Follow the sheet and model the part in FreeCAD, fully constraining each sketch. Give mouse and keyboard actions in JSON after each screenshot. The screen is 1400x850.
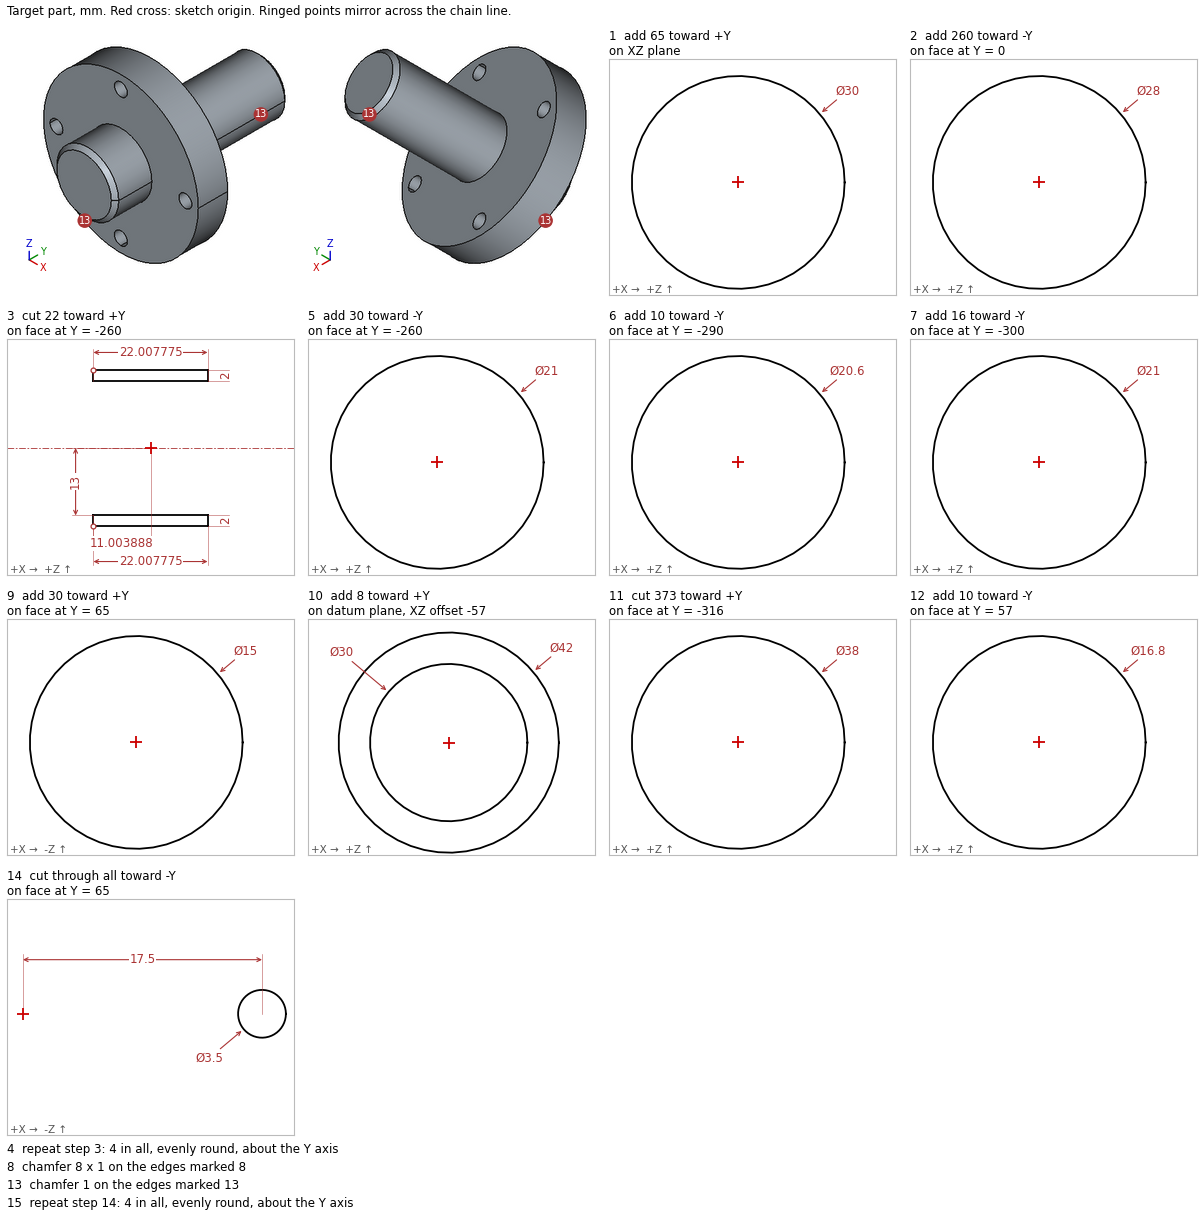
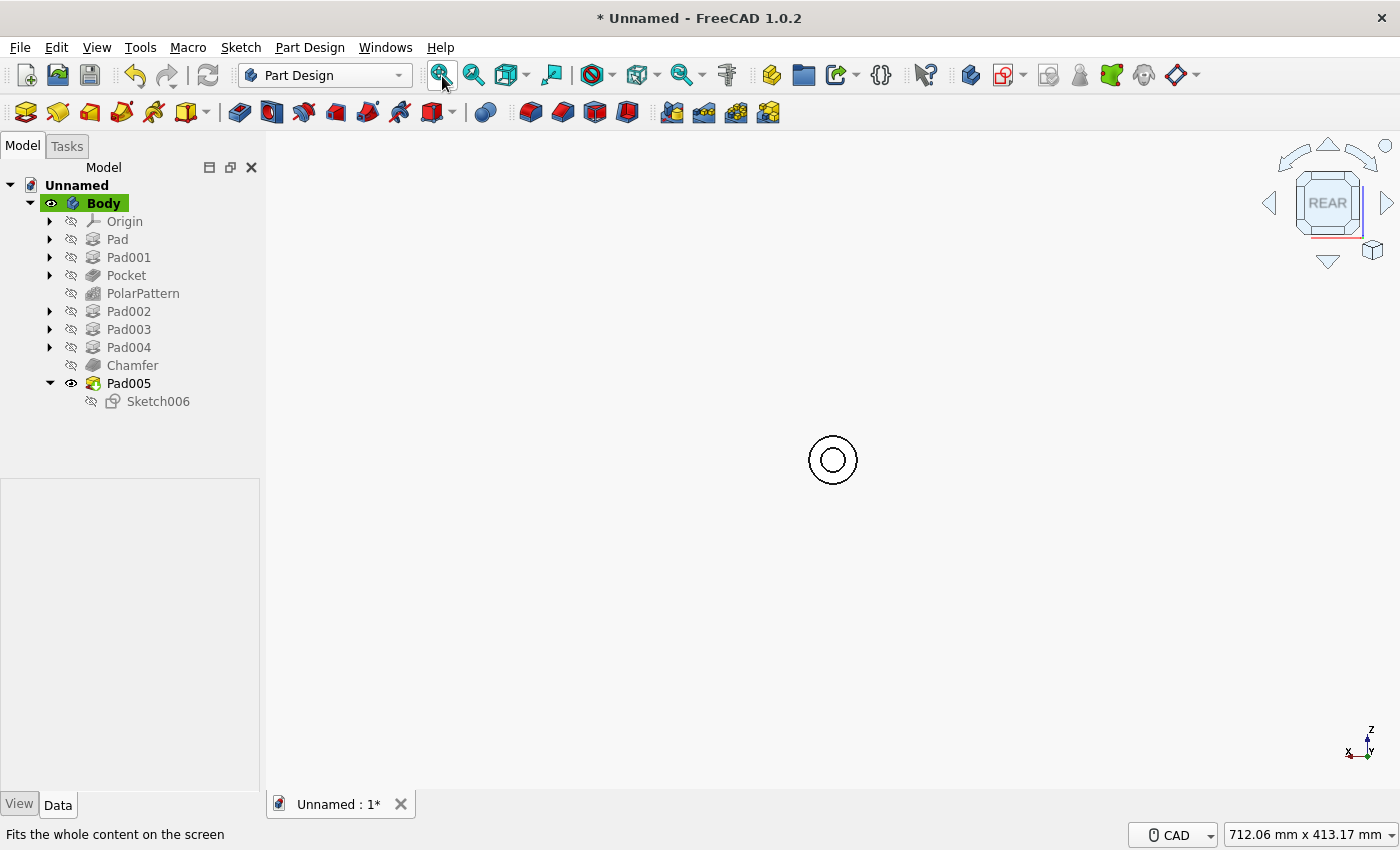
{"action": "left_click", "coordinate": [50, 221]}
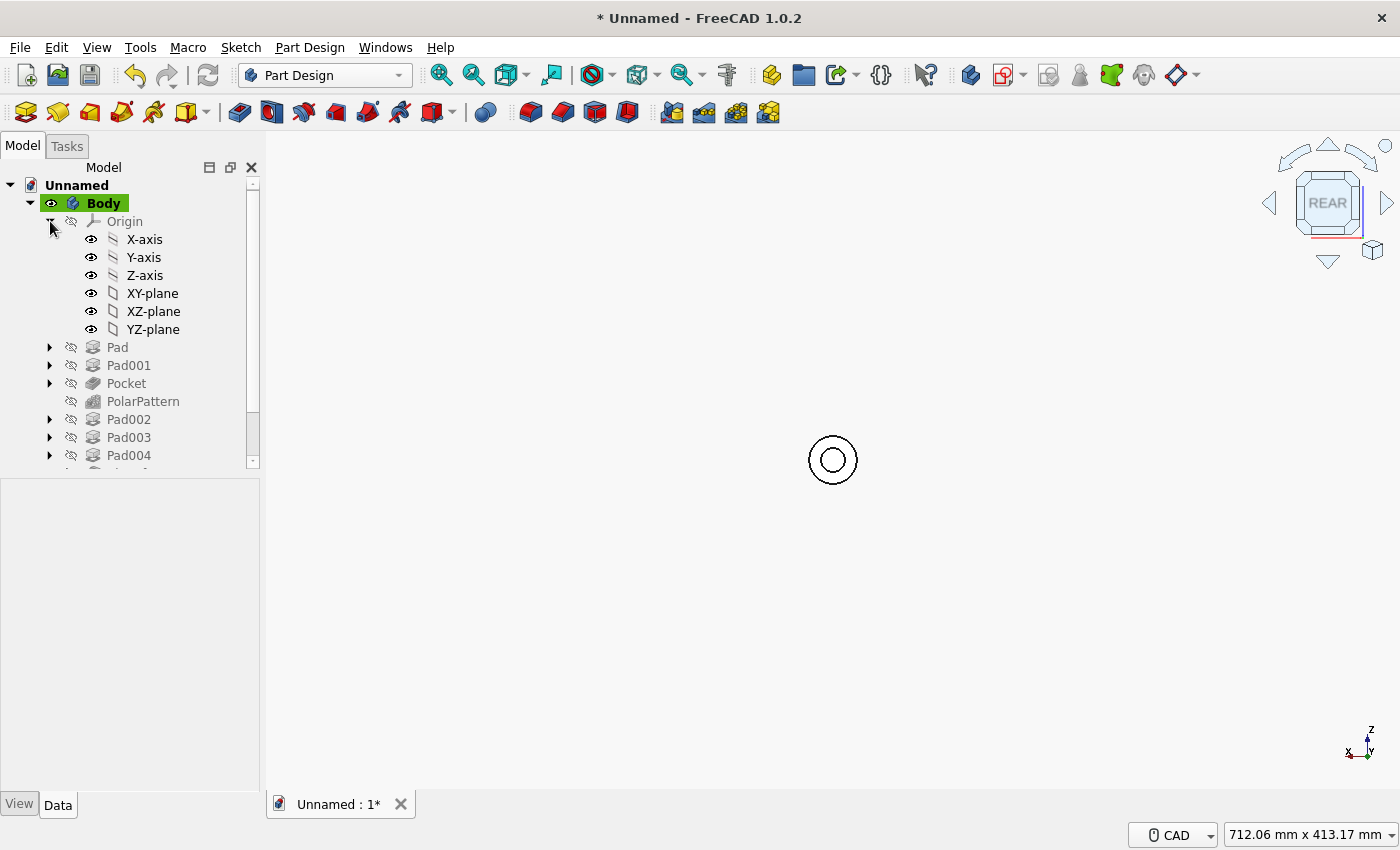
{"action": "left_click", "coordinate": [136, 311]}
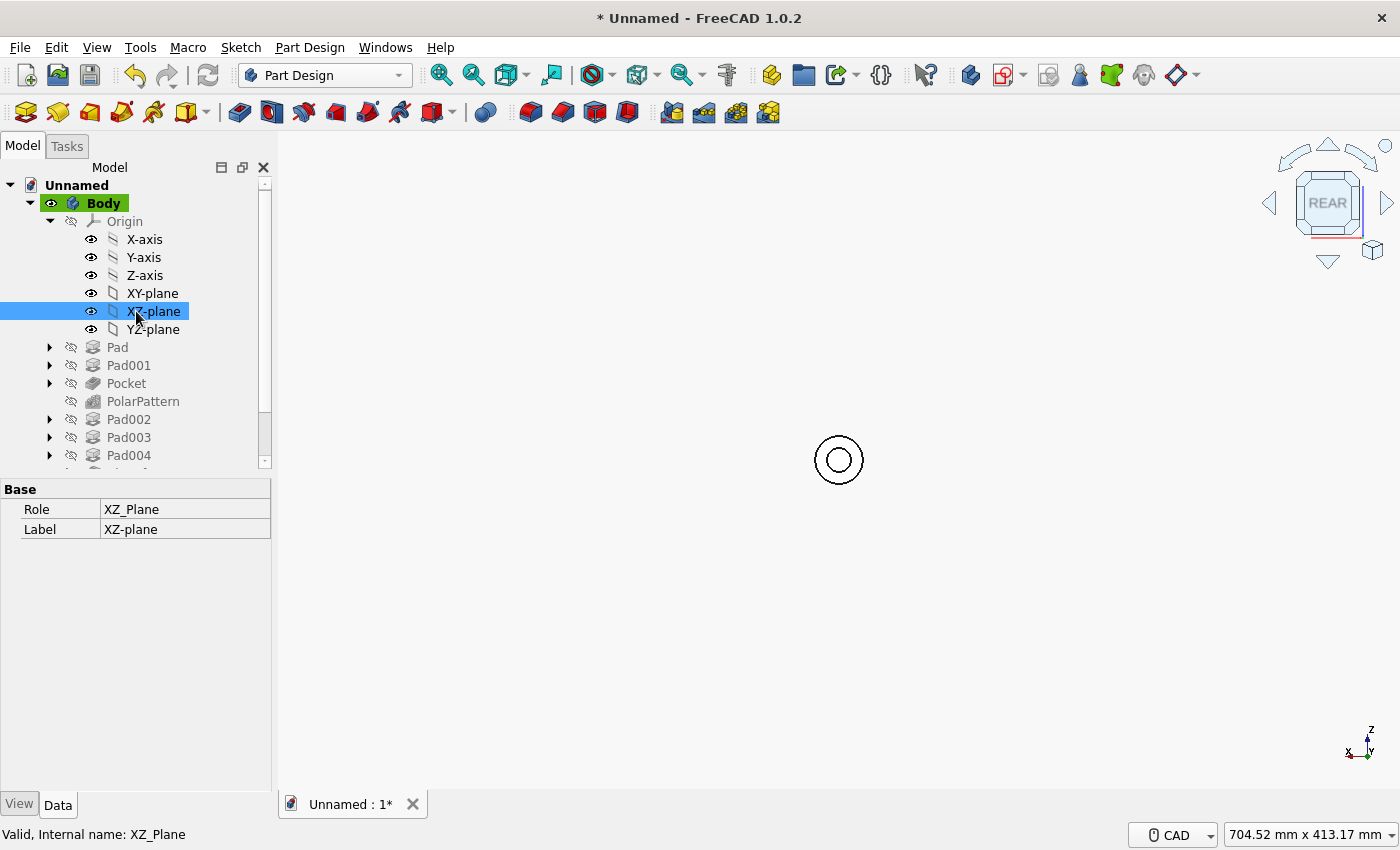
{"action": "left_click", "coordinate": [1176, 76]}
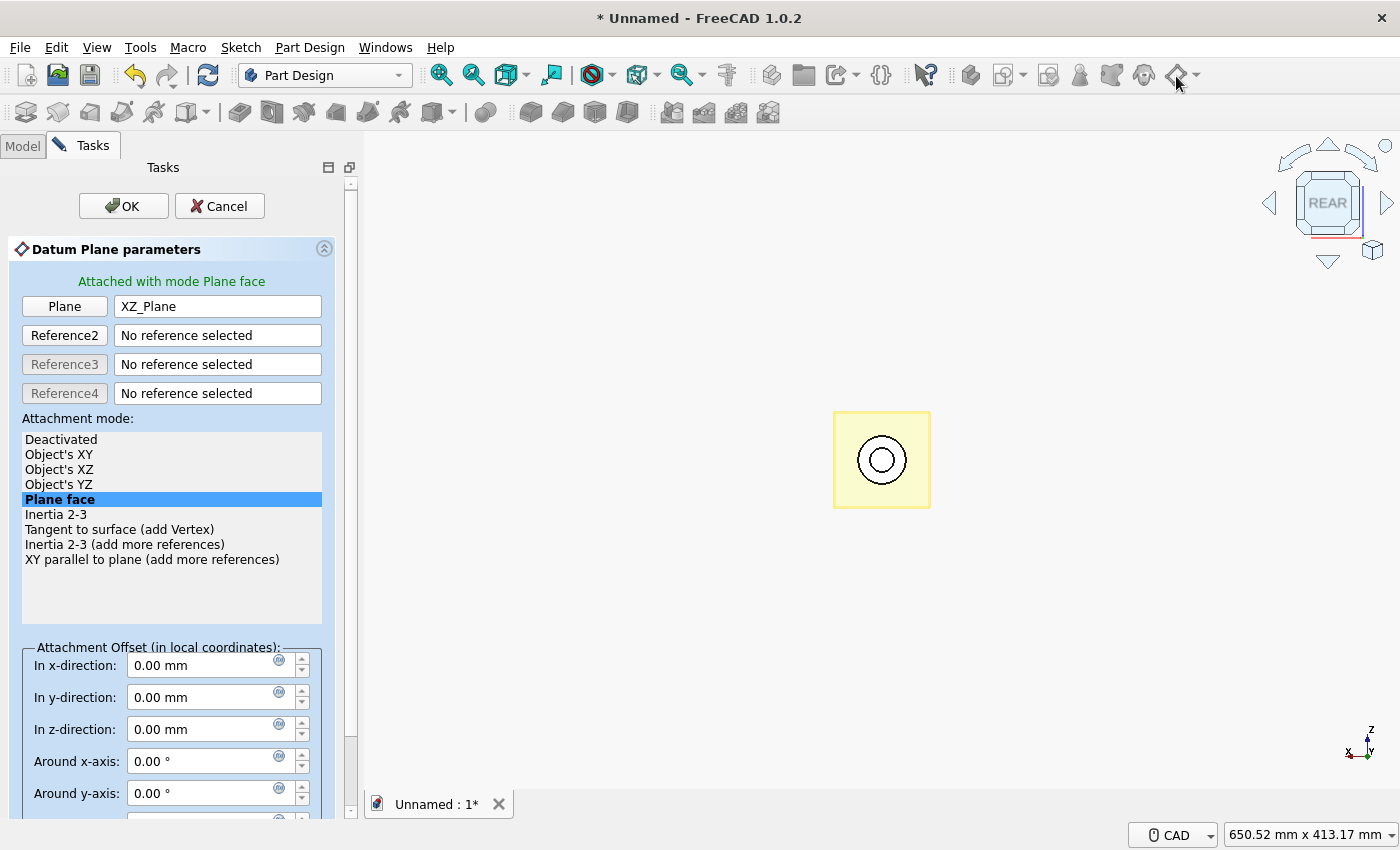
{"action": "triple_click", "coordinate": [210, 729]}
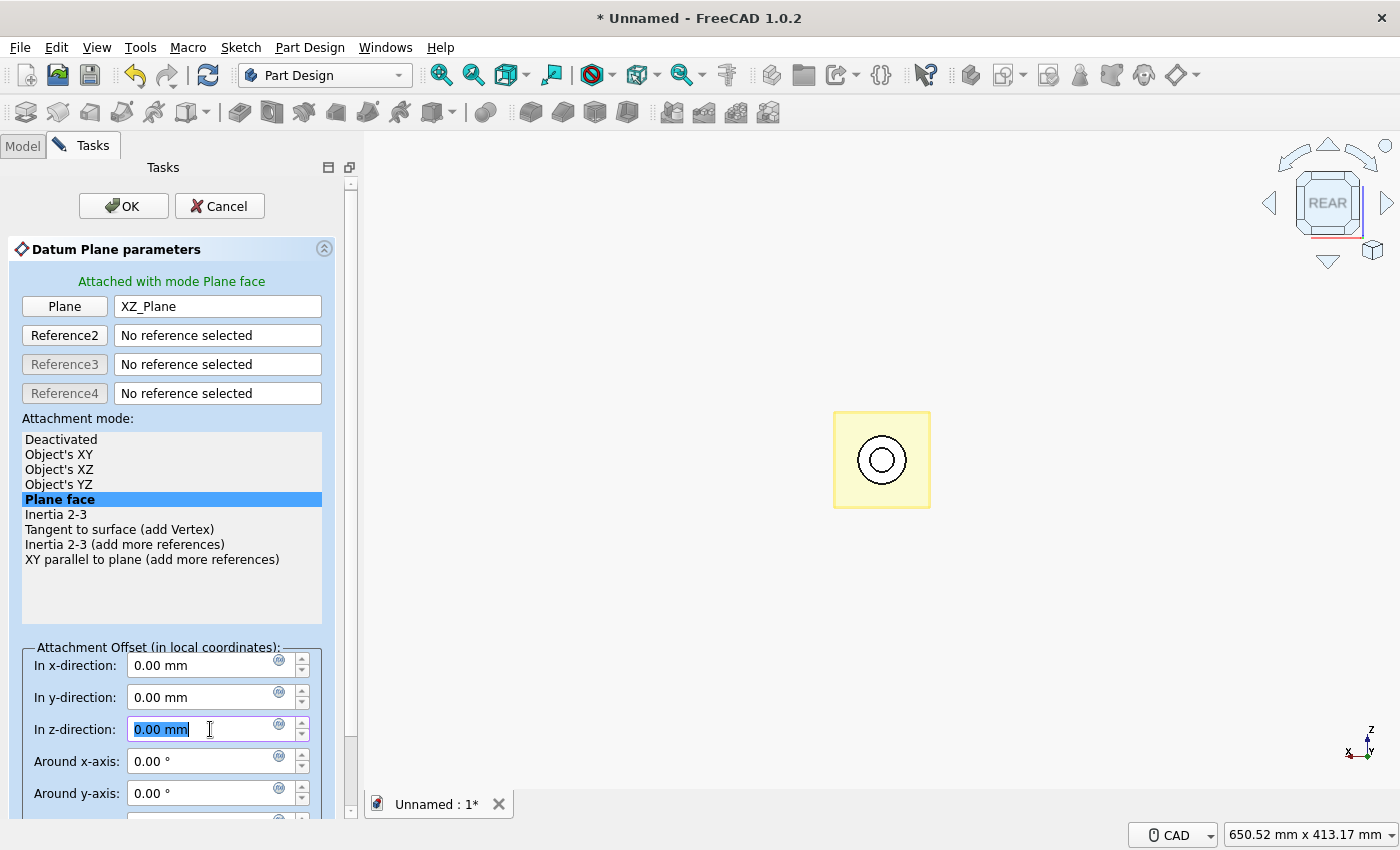
{"action": "type", "text": "-57"}
{"action": "key", "text": "Tab"}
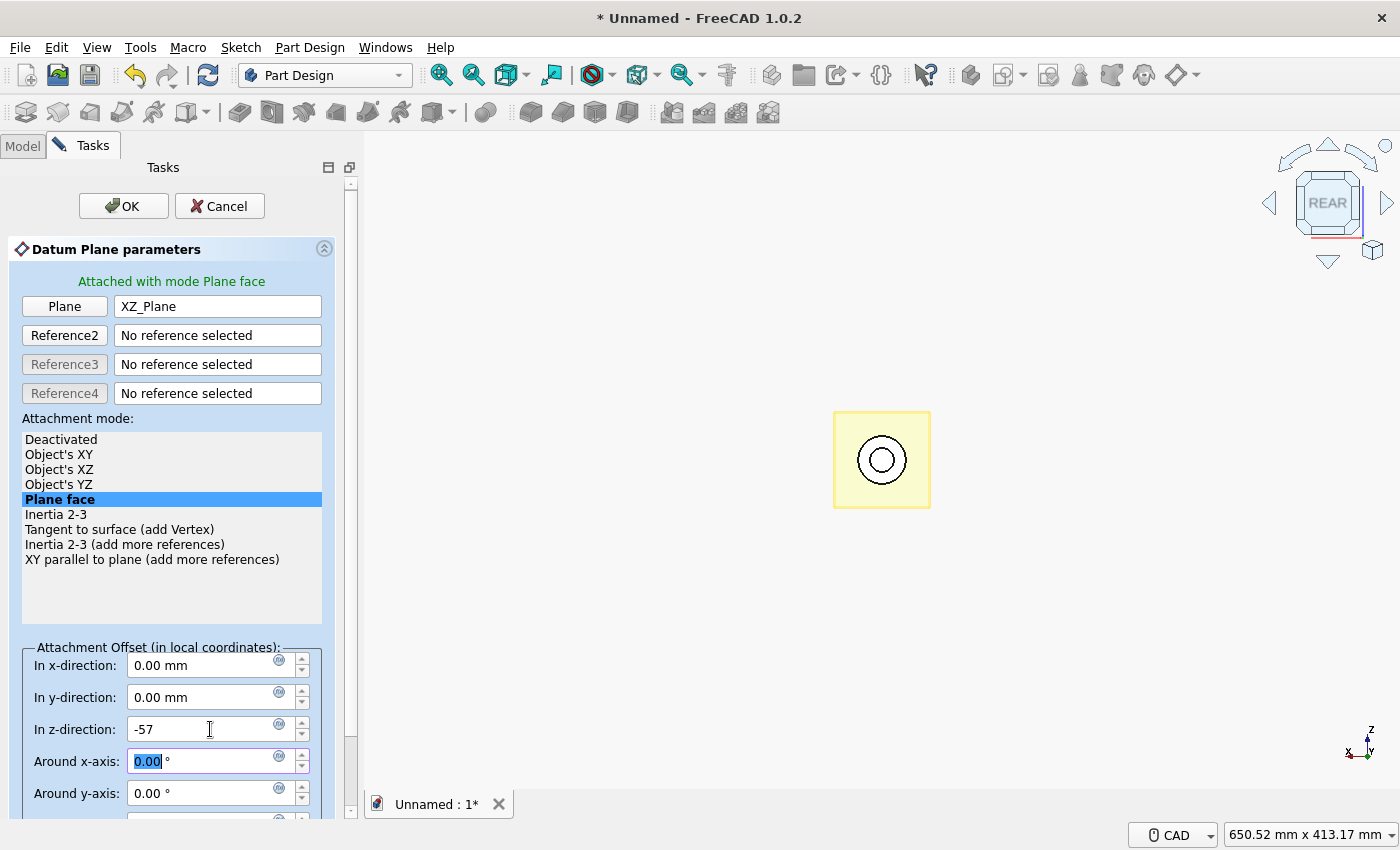
{"action": "left_click", "coordinate": [124, 206]}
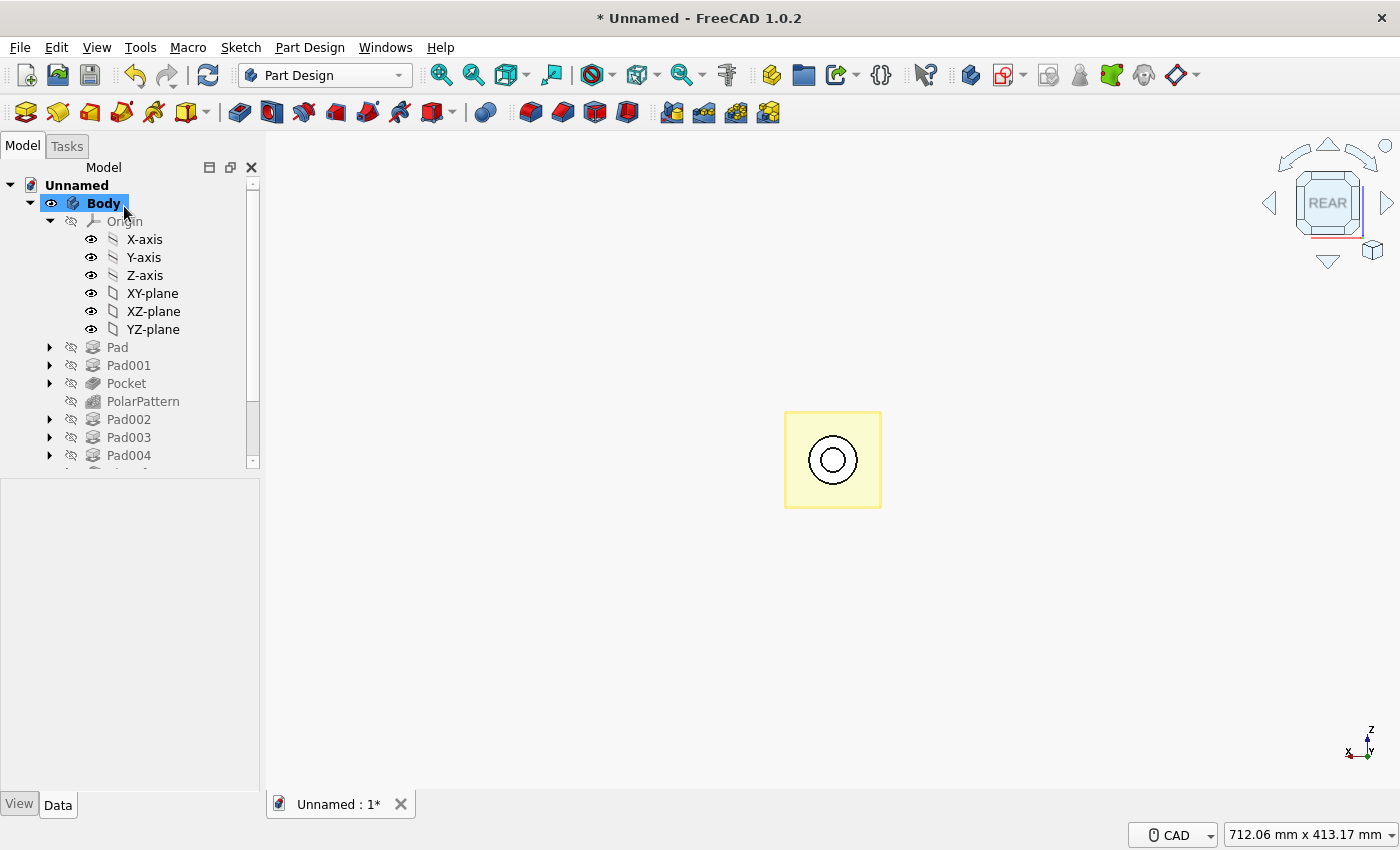
{"action": "scroll", "coordinate": [100, 325], "scroll_direction": "down", "scroll_amount": 3}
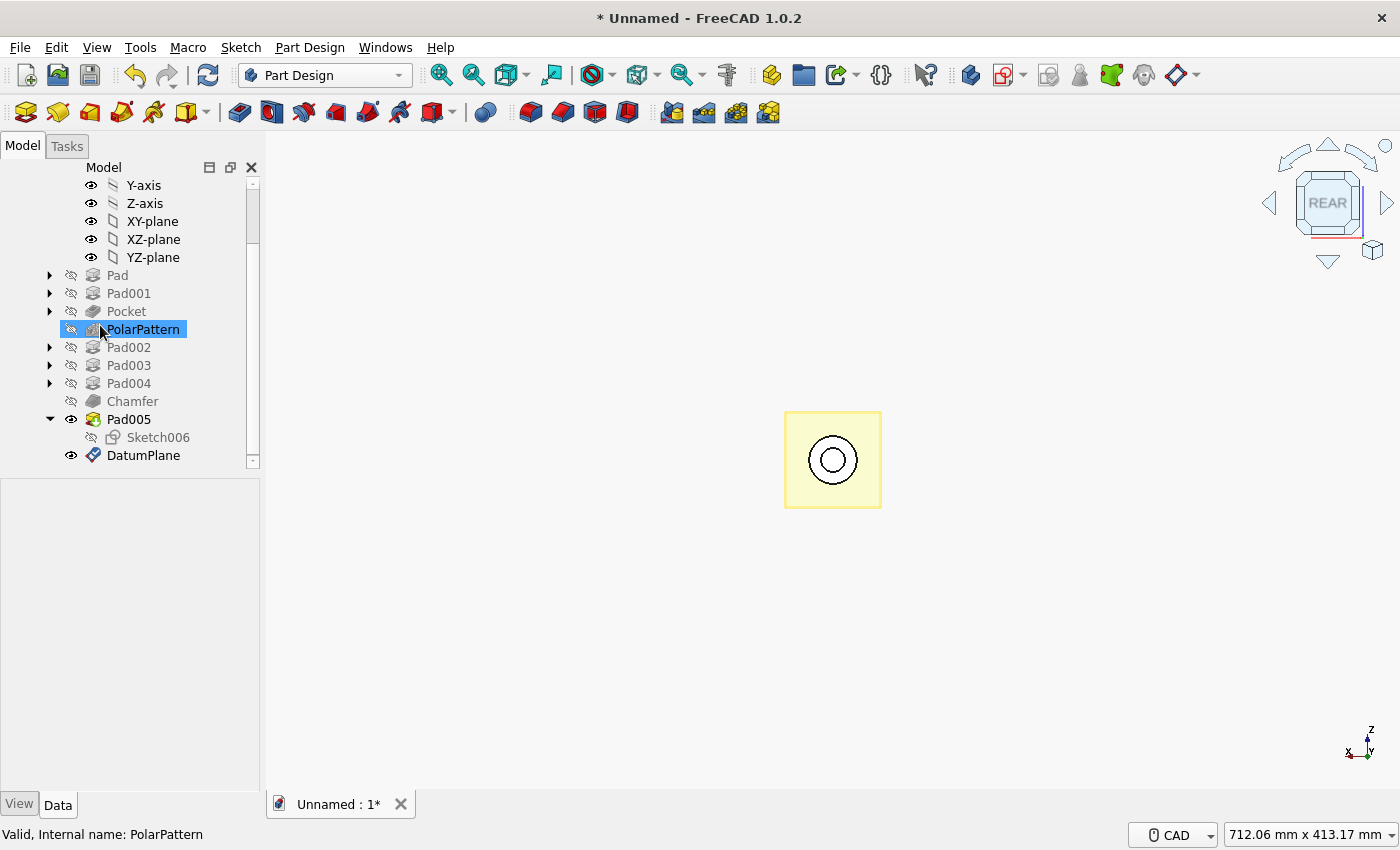
{"action": "left_click", "coordinate": [116, 455]}